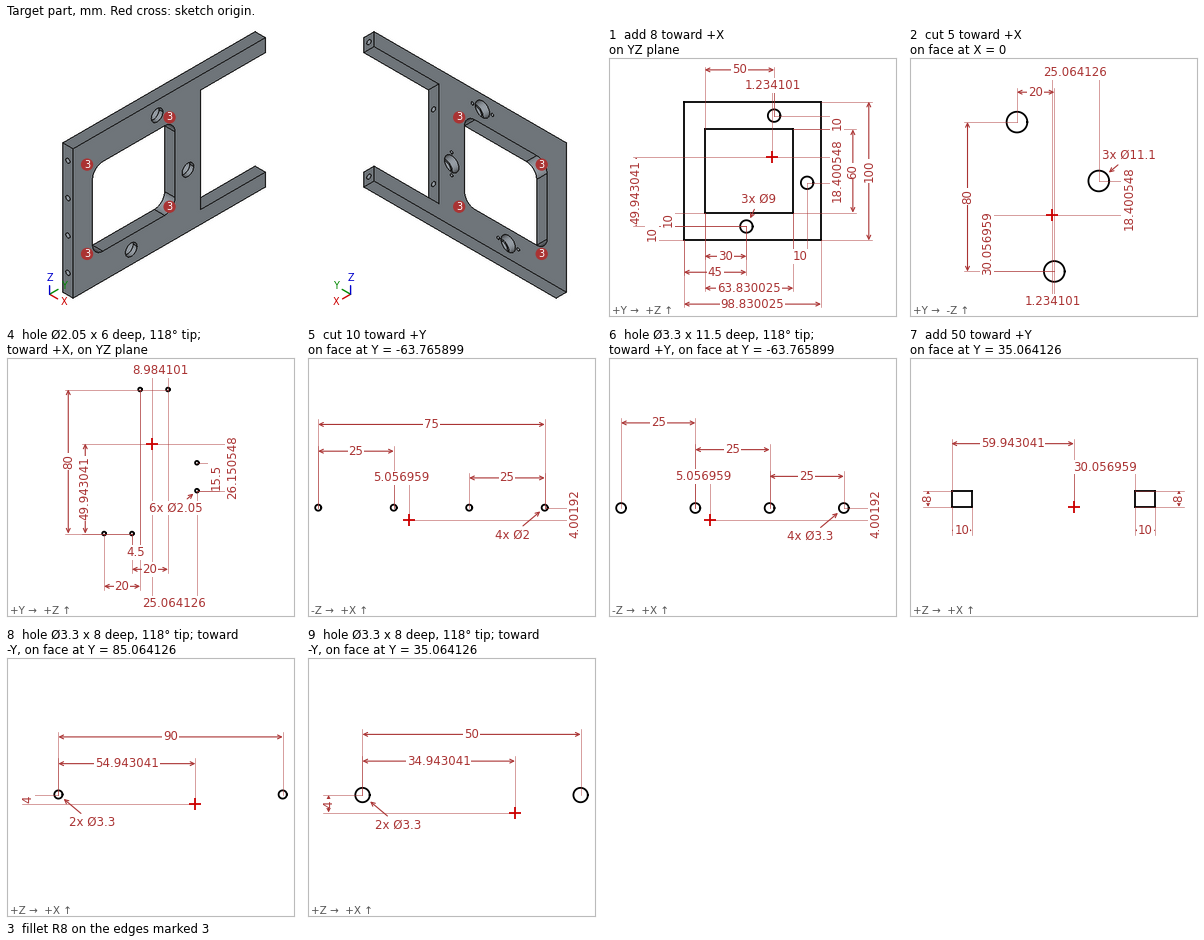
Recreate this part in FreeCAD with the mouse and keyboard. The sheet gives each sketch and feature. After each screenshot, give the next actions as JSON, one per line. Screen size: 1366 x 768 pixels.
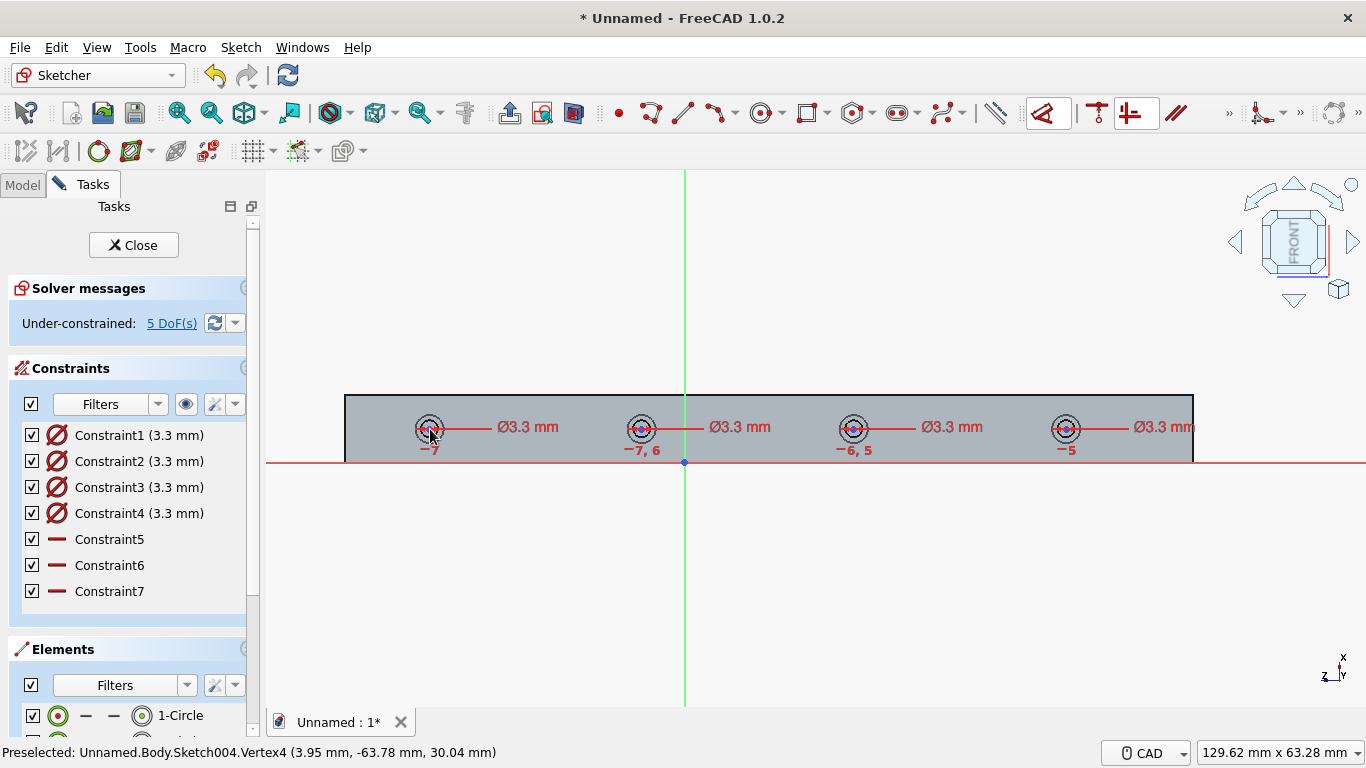
{"action": "left_click", "coordinate": [1066, 429]}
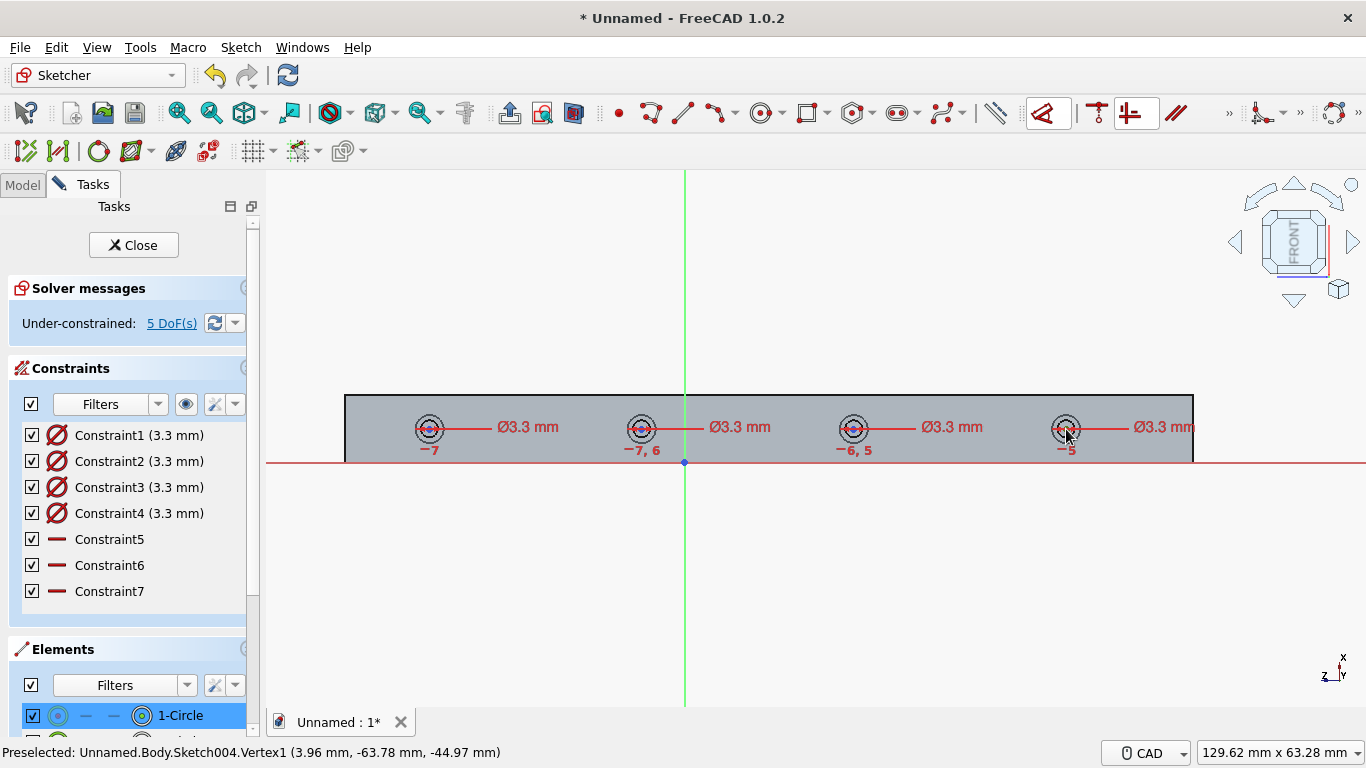
{"action": "left_click", "coordinate": [854, 429]}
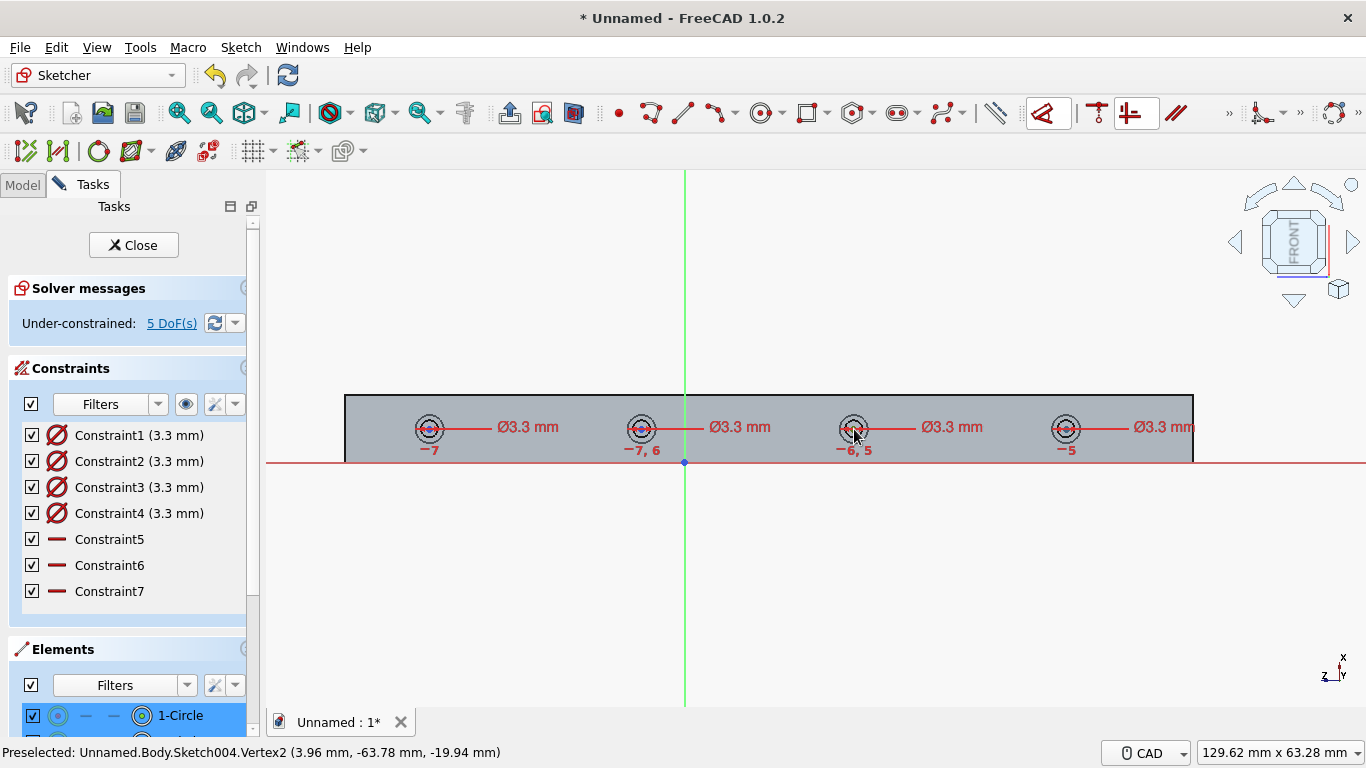
{"action": "left_click", "coordinate": [1066, 114]}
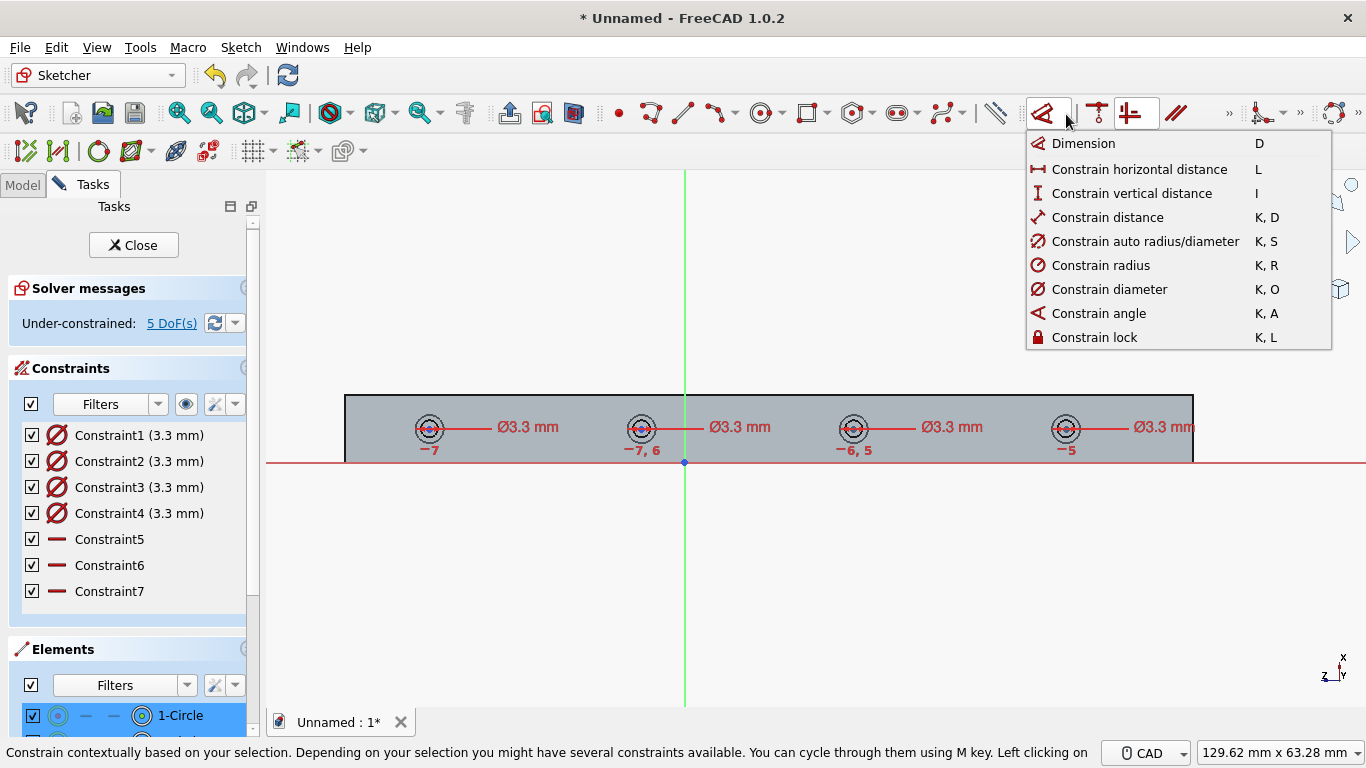
{"action": "left_click", "coordinate": [1179, 169]}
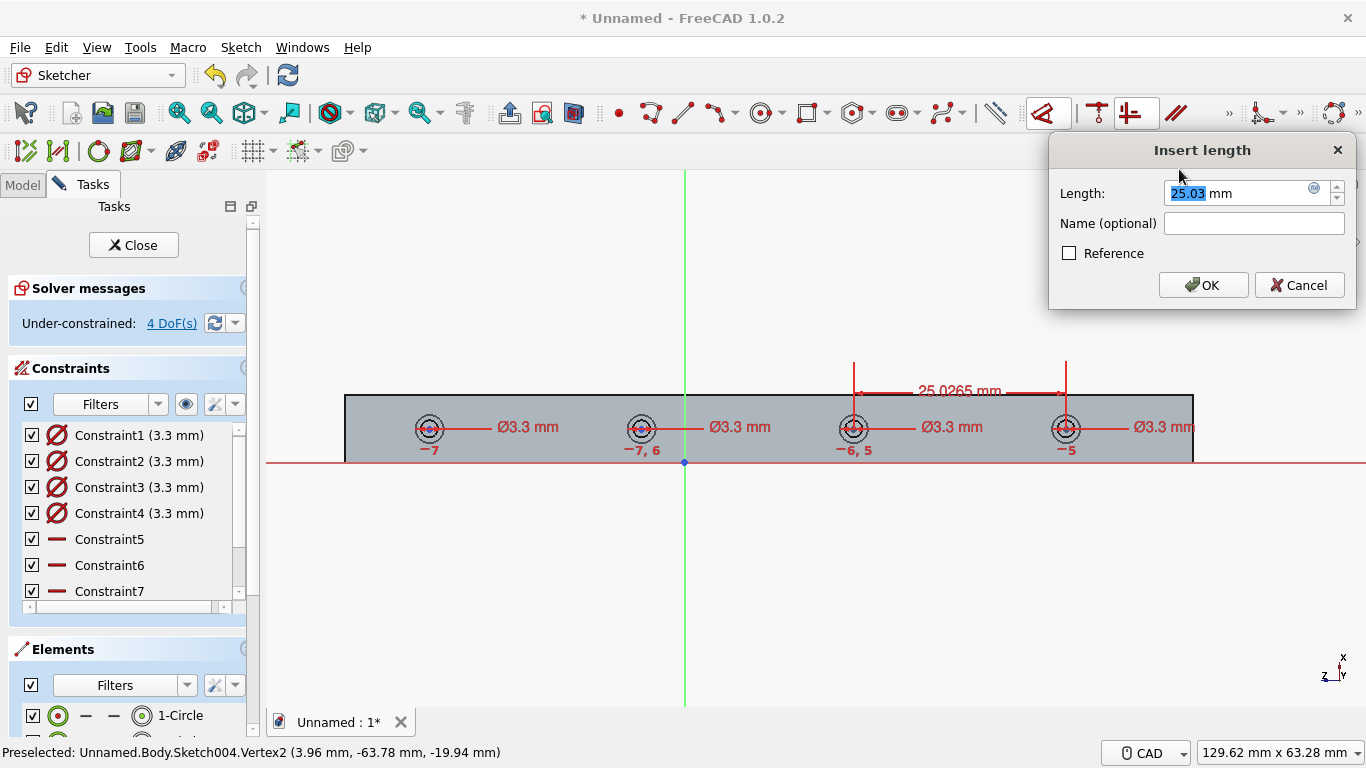
{"action": "type", "text": "25"}
{"action": "key", "text": "Return"}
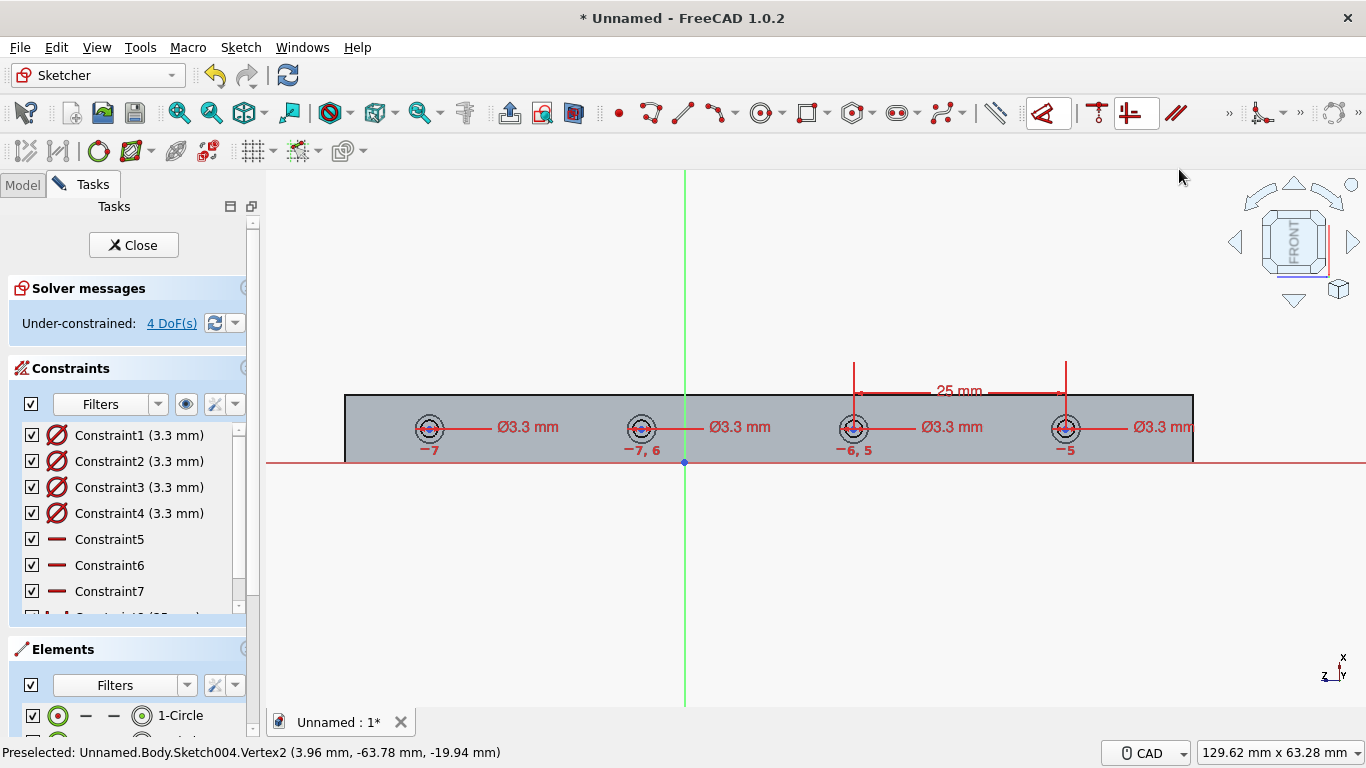
{"action": "left_click", "coordinate": [854, 429]}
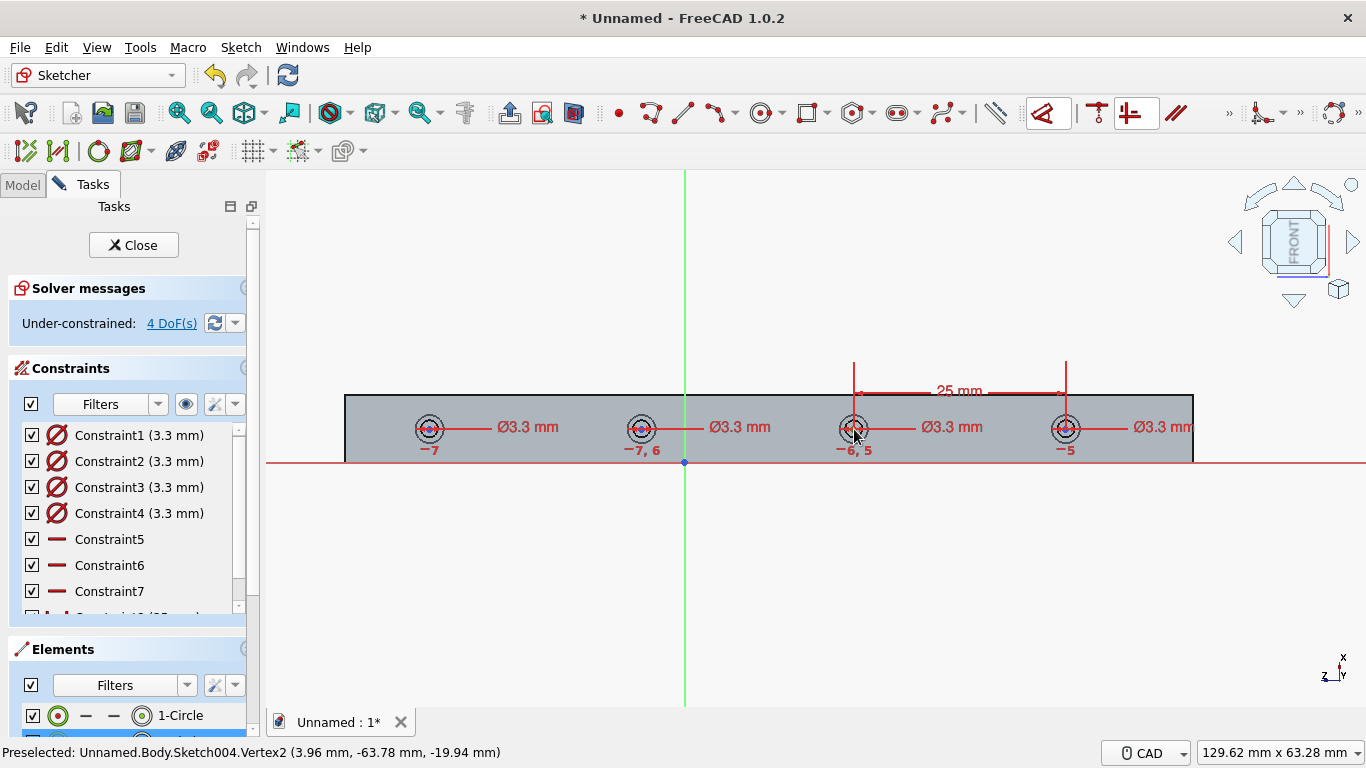
{"action": "left_click", "coordinate": [642, 429]}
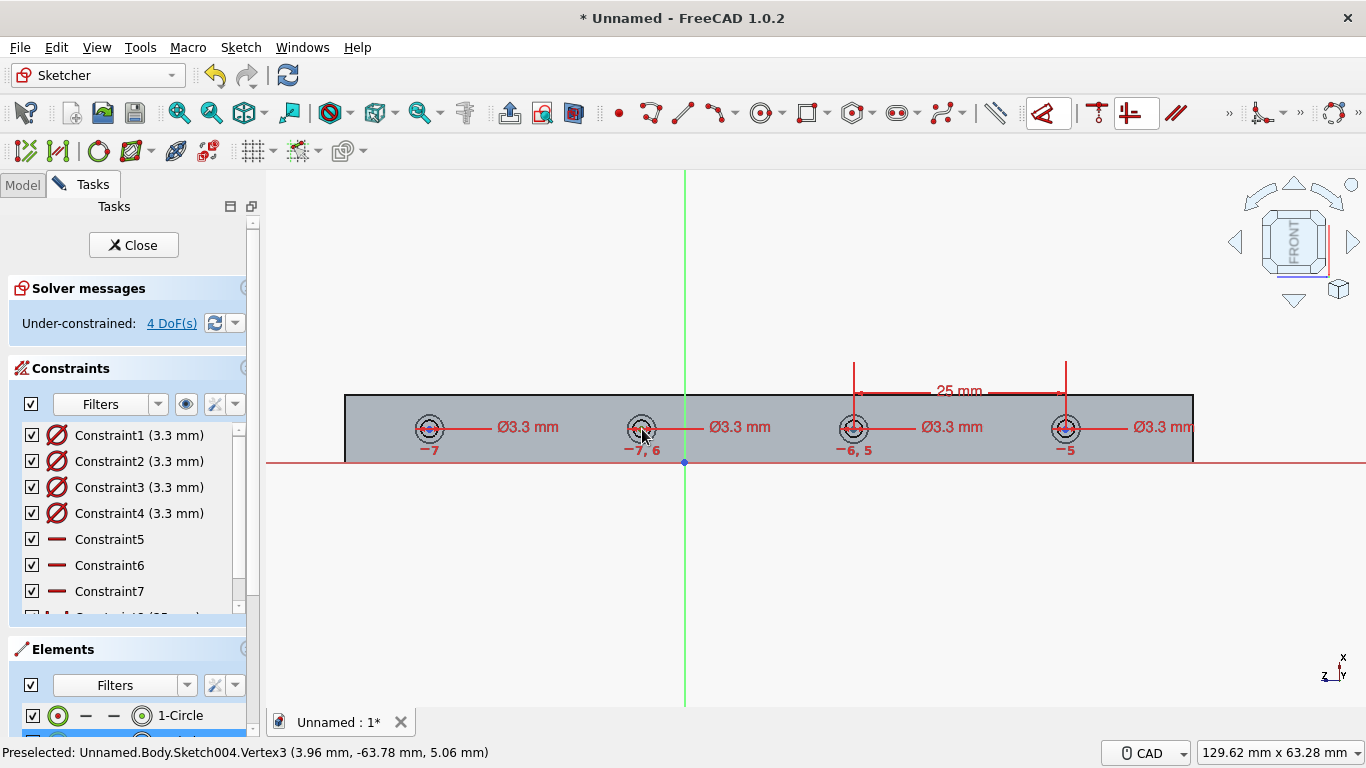
{"action": "left_click", "coordinate": [1066, 114]}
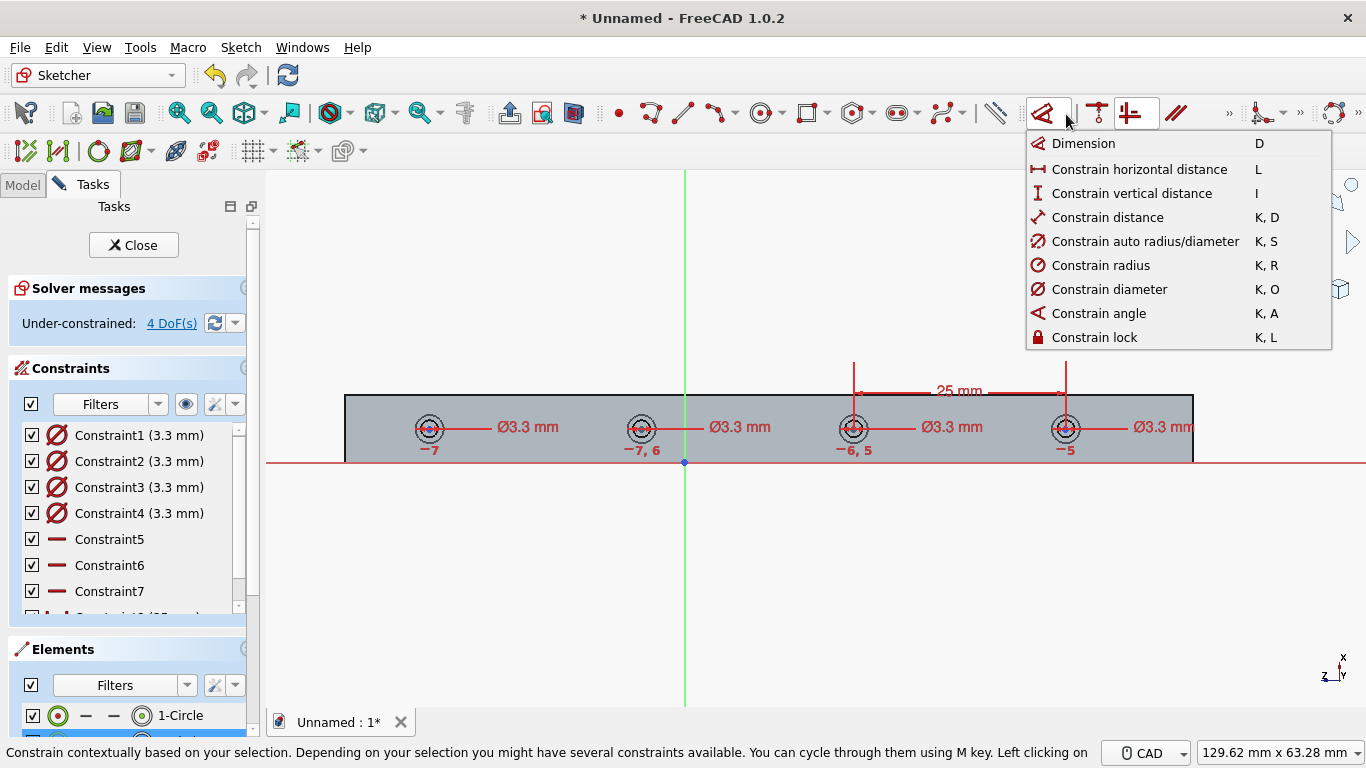
{"action": "left_click", "coordinate": [1179, 169]}